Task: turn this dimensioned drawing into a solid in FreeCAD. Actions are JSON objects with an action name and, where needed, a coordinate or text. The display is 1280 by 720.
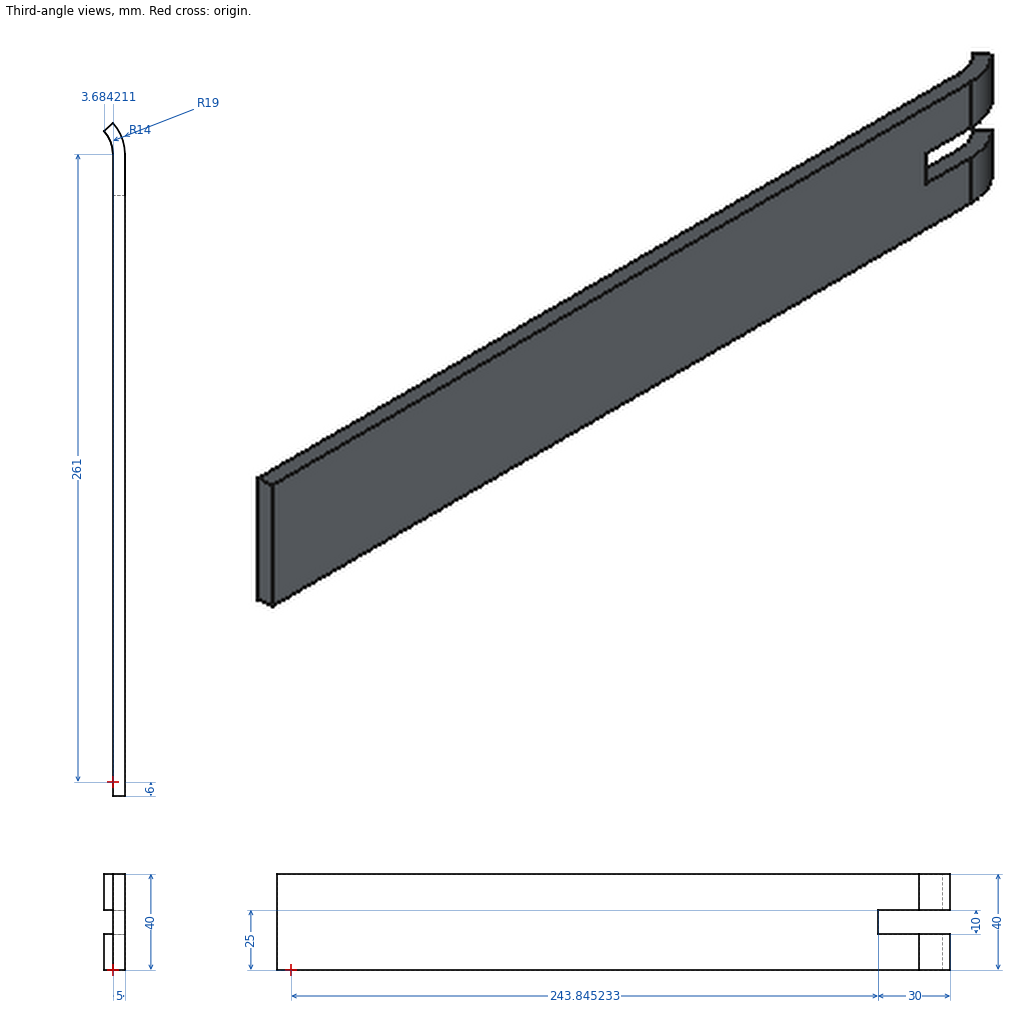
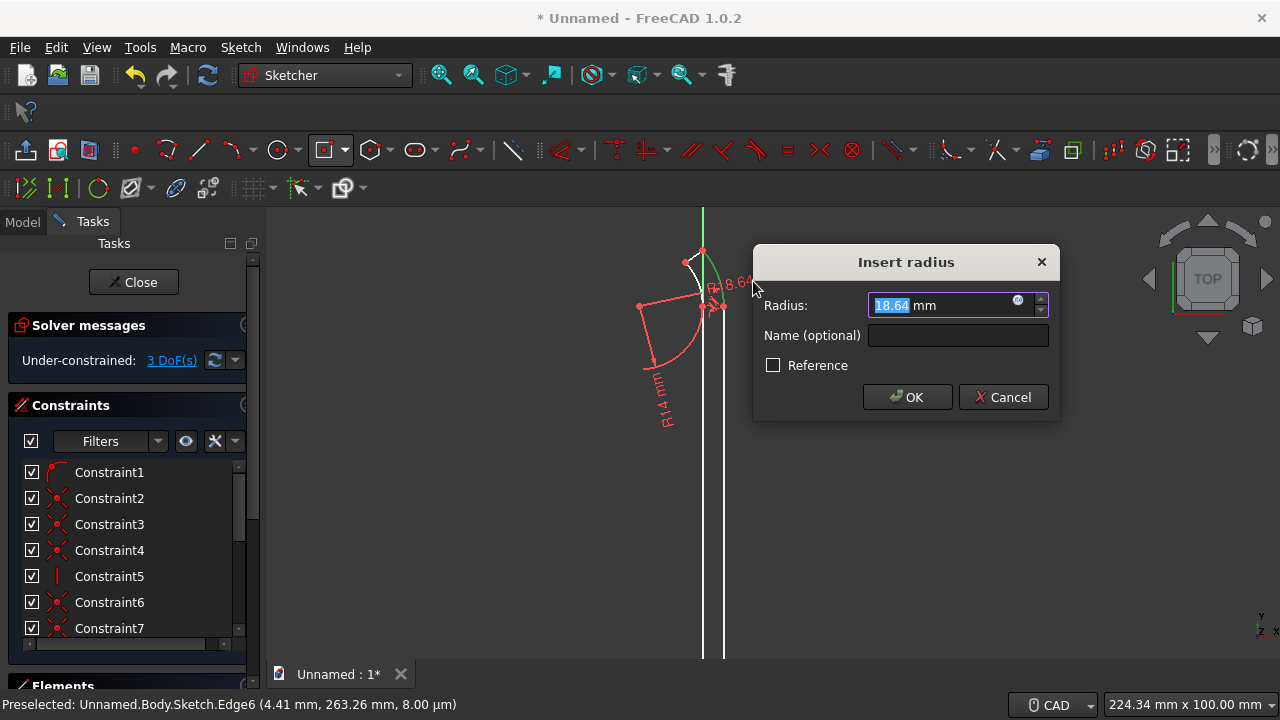
{"action": "type", "text": "19"}
{"action": "key", "text": "Return"}
{"action": "key", "text": "Escape"}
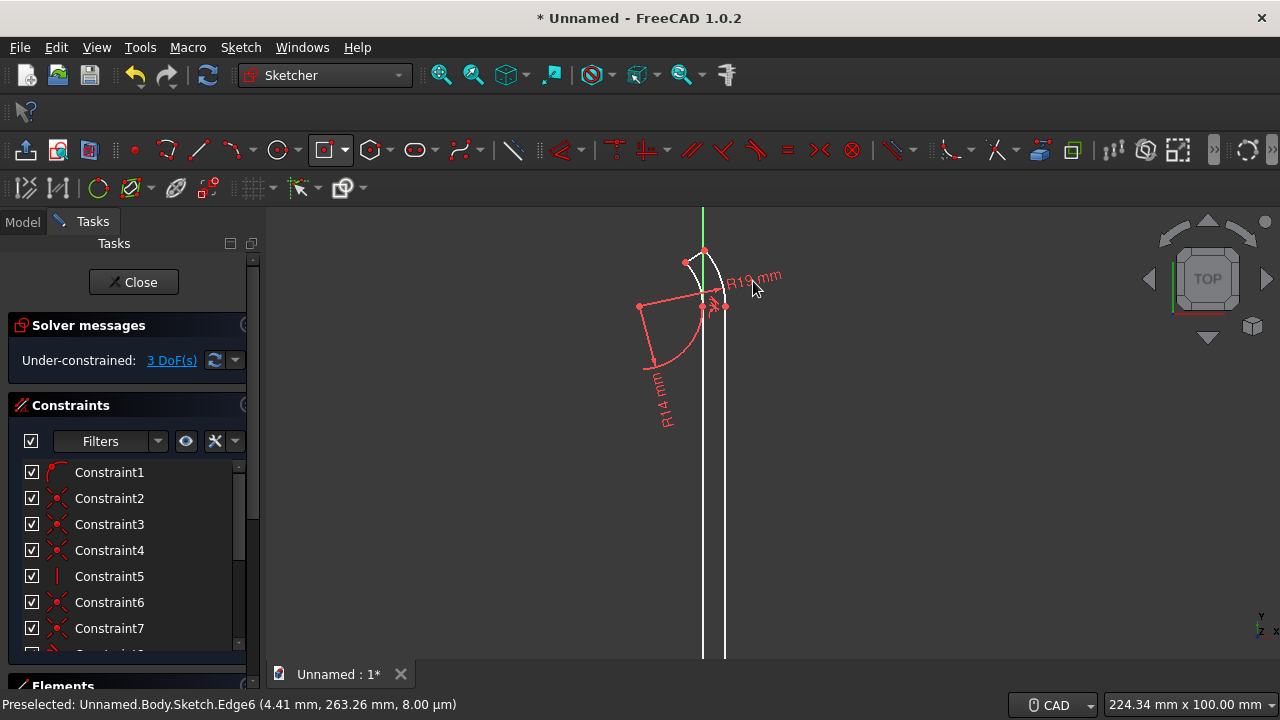
{"action": "left_click", "coordinate": [705, 250]}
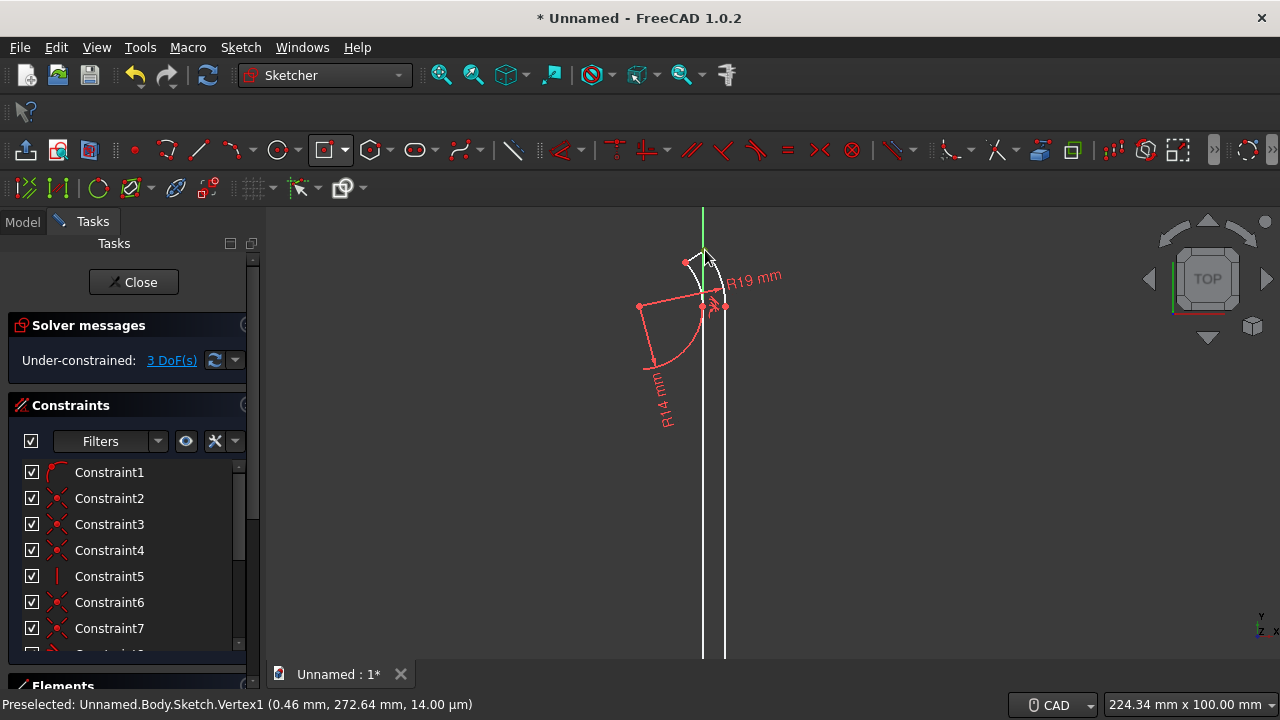
{"action": "left_click", "coordinate": [703, 263]}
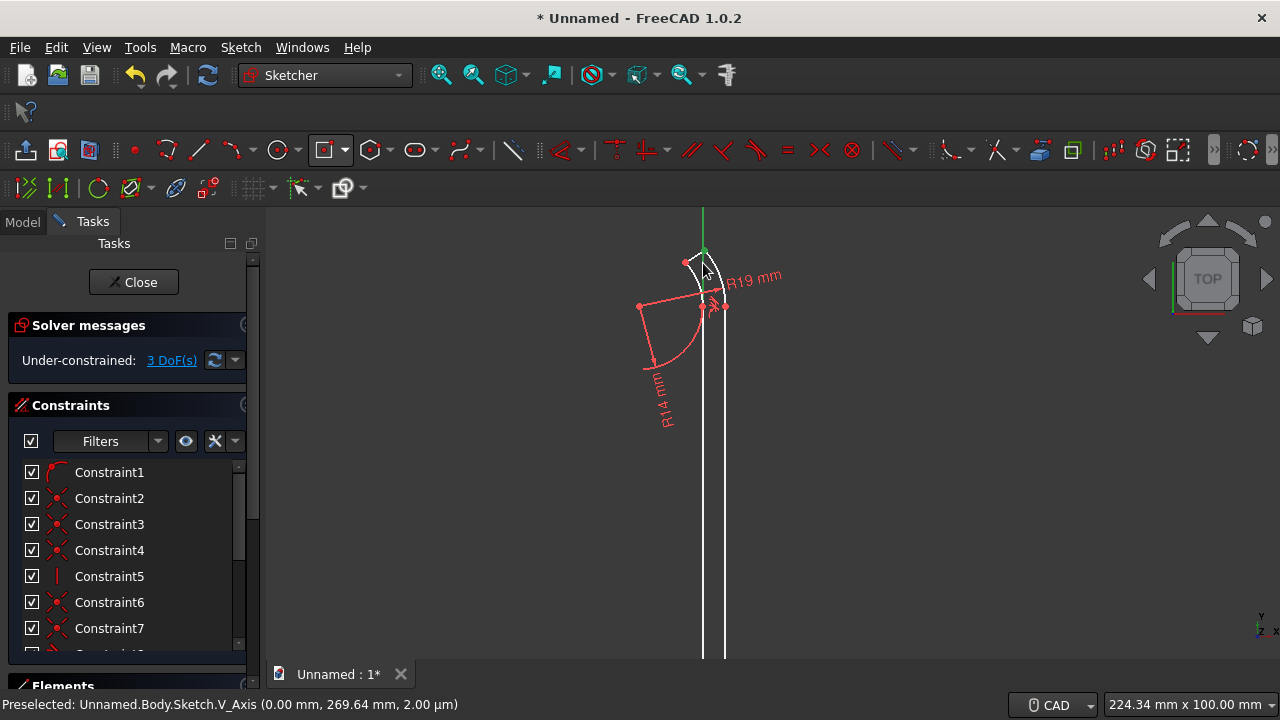
{"action": "left_click", "coordinate": [616, 150]}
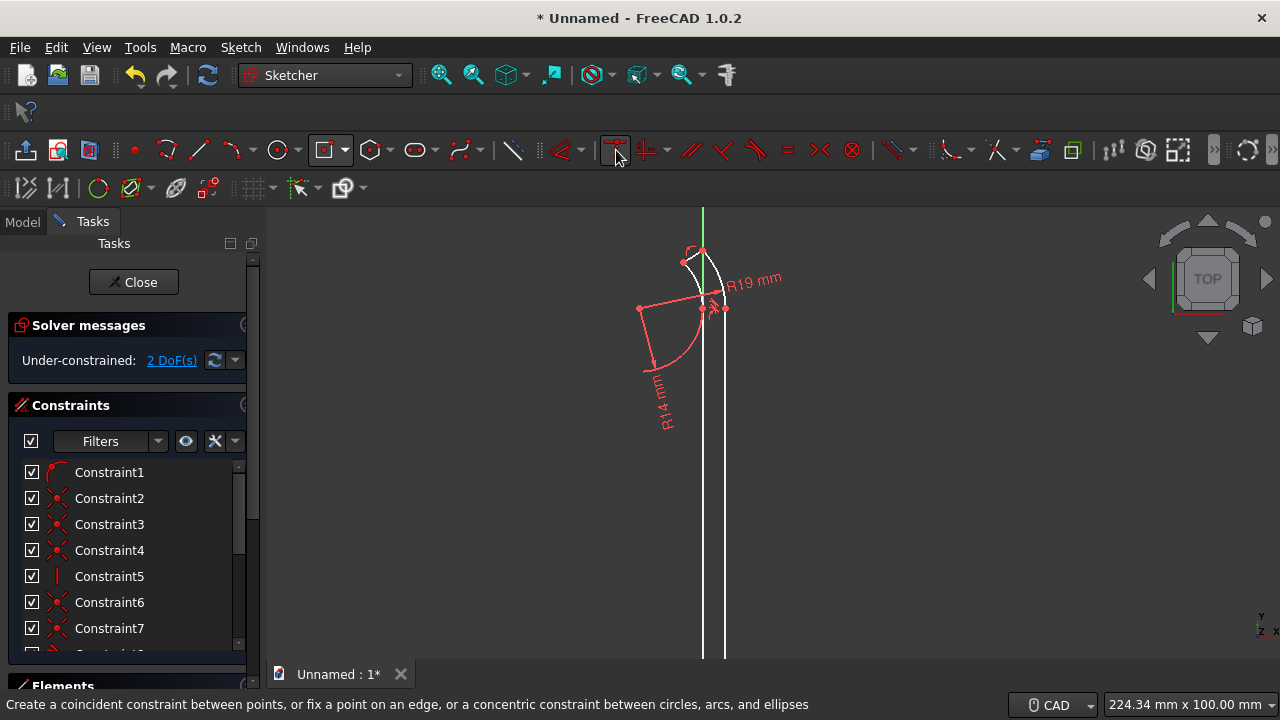
{"action": "left_click", "coordinate": [560, 150]}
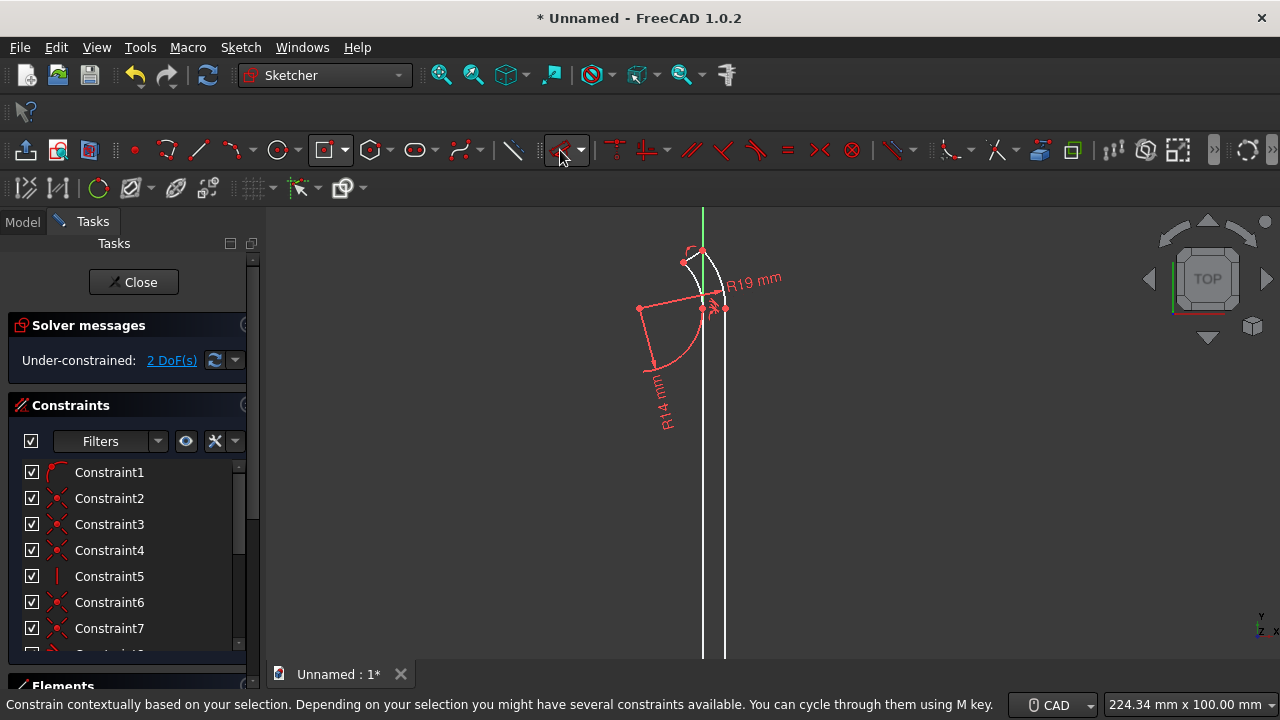
{"action": "left_click", "coordinate": [703, 543]}
{"action": "left_click", "coordinate": [669, 470]}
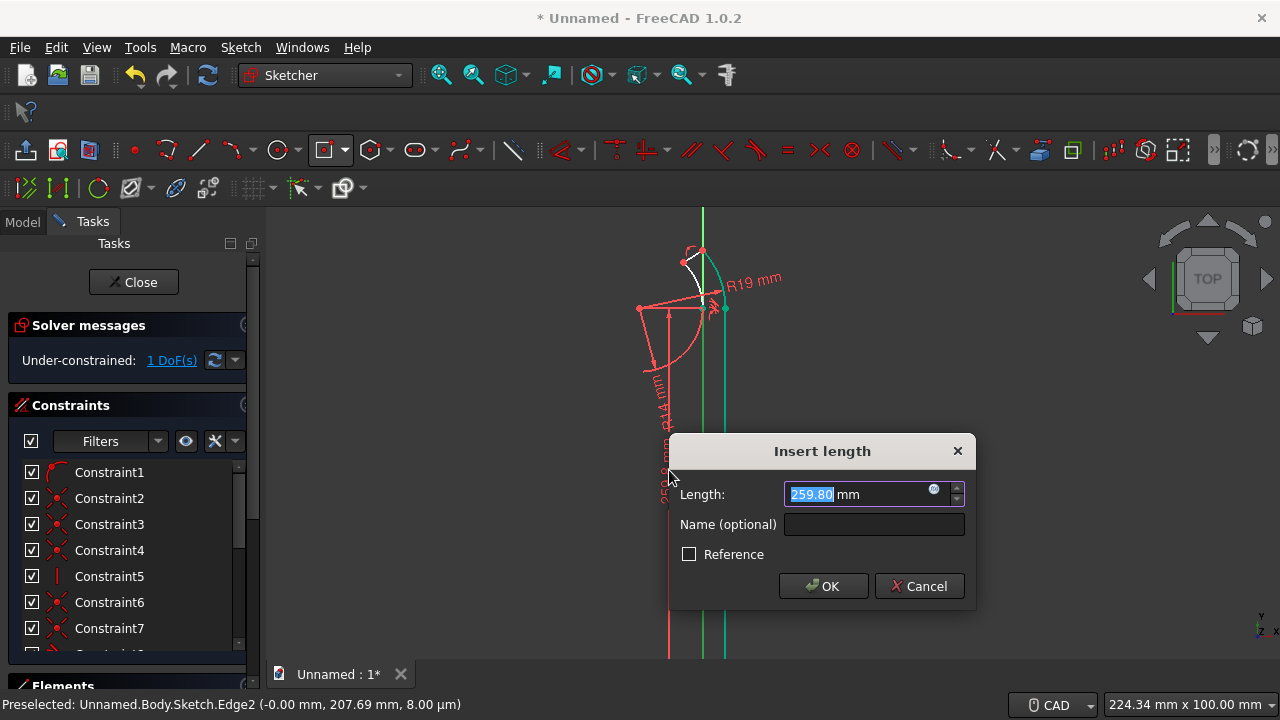
{"action": "type", "text": "261"}
{"action": "key", "text": "Return"}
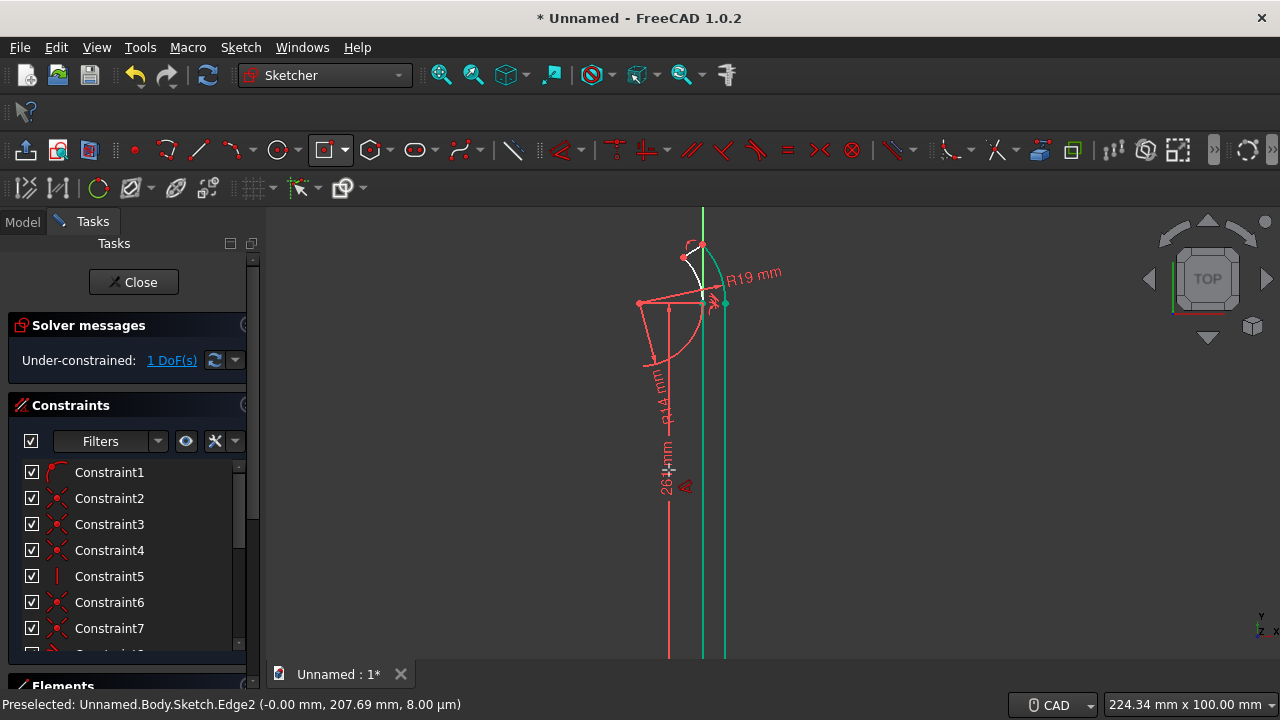
{"action": "scroll", "coordinate": [683, 257], "scroll_direction": "up", "scroll_amount": 5}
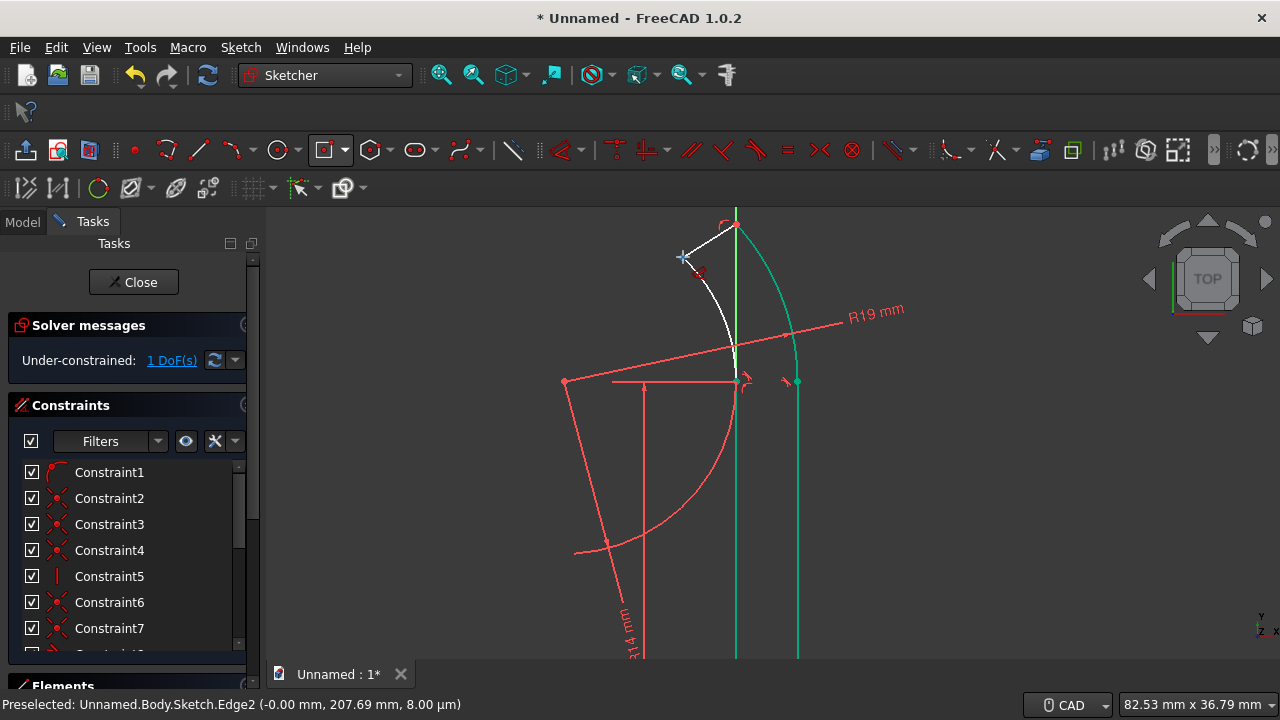
{"action": "left_click", "coordinate": [683, 258]}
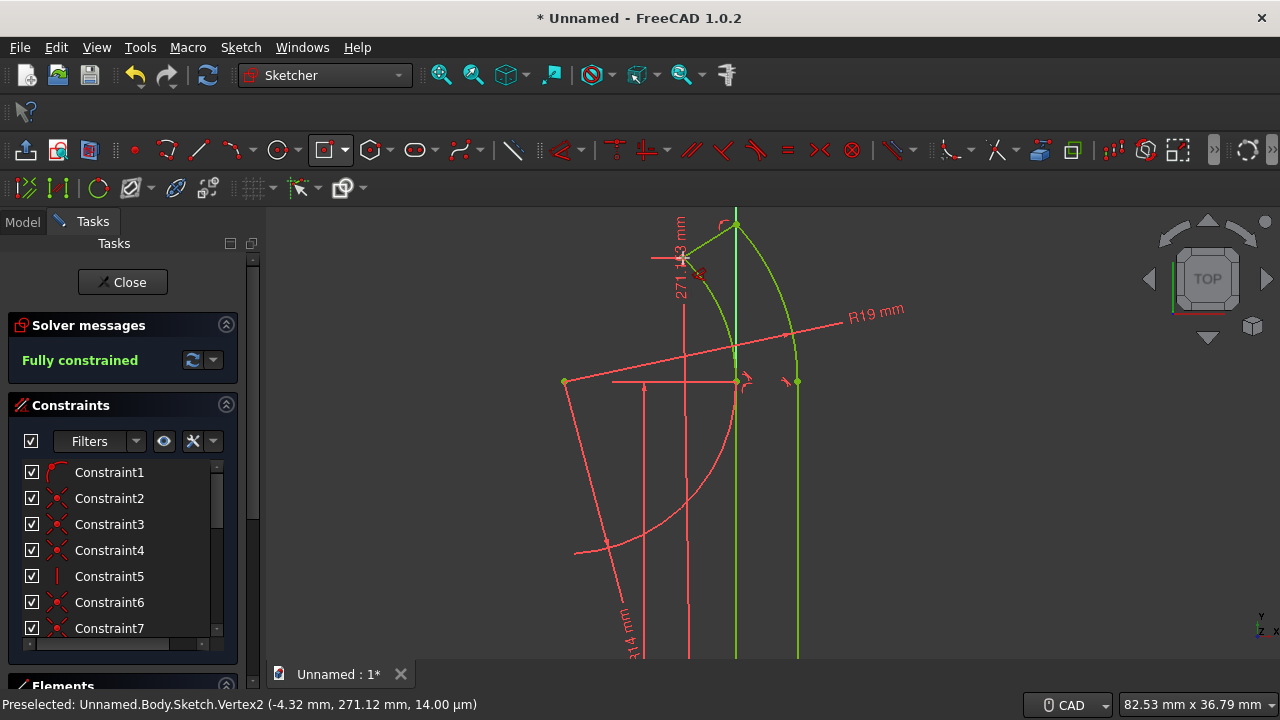
{"action": "key", "text": "Escape"}
{"action": "key", "text": "Escape"}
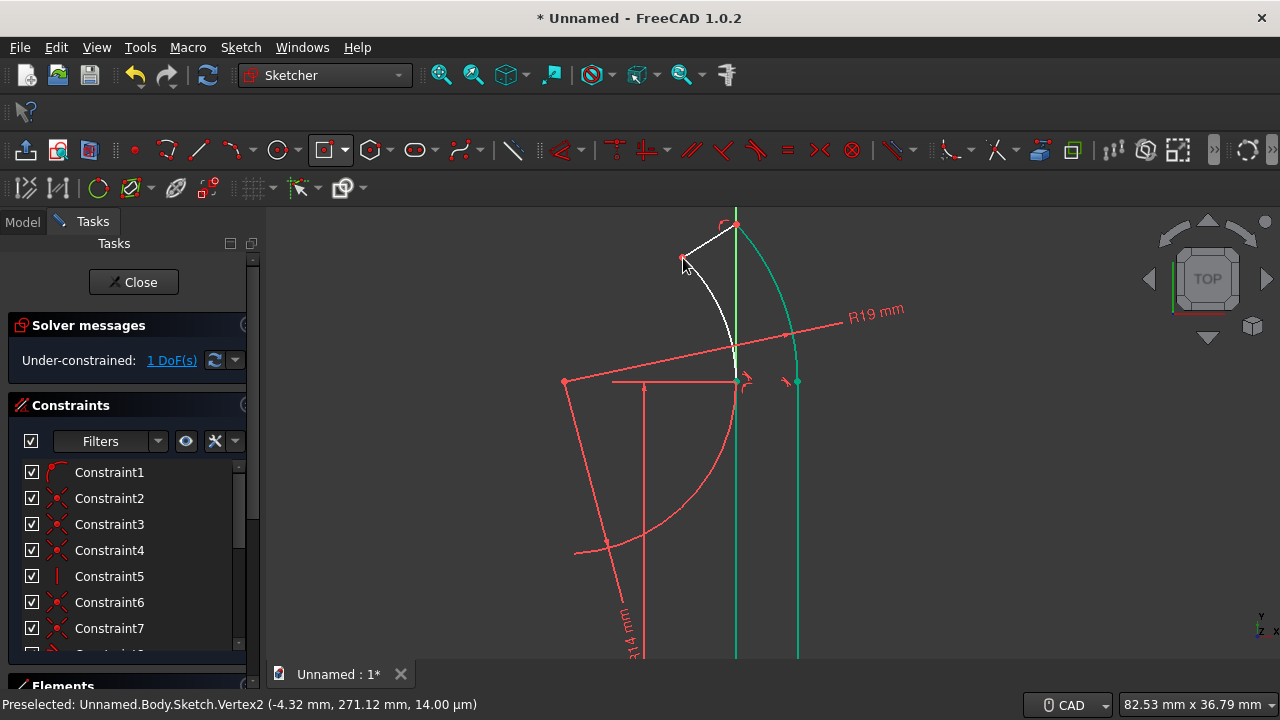
{"action": "left_click", "coordinate": [683, 258]}